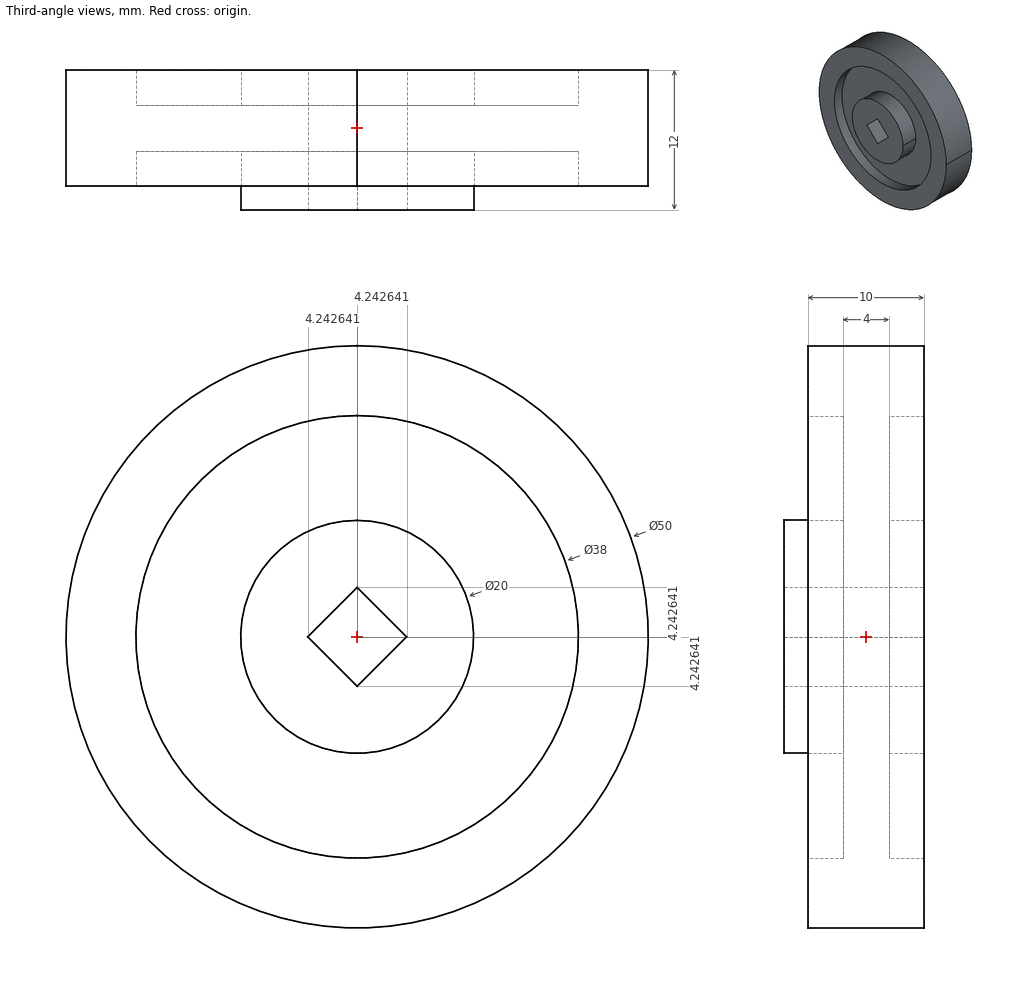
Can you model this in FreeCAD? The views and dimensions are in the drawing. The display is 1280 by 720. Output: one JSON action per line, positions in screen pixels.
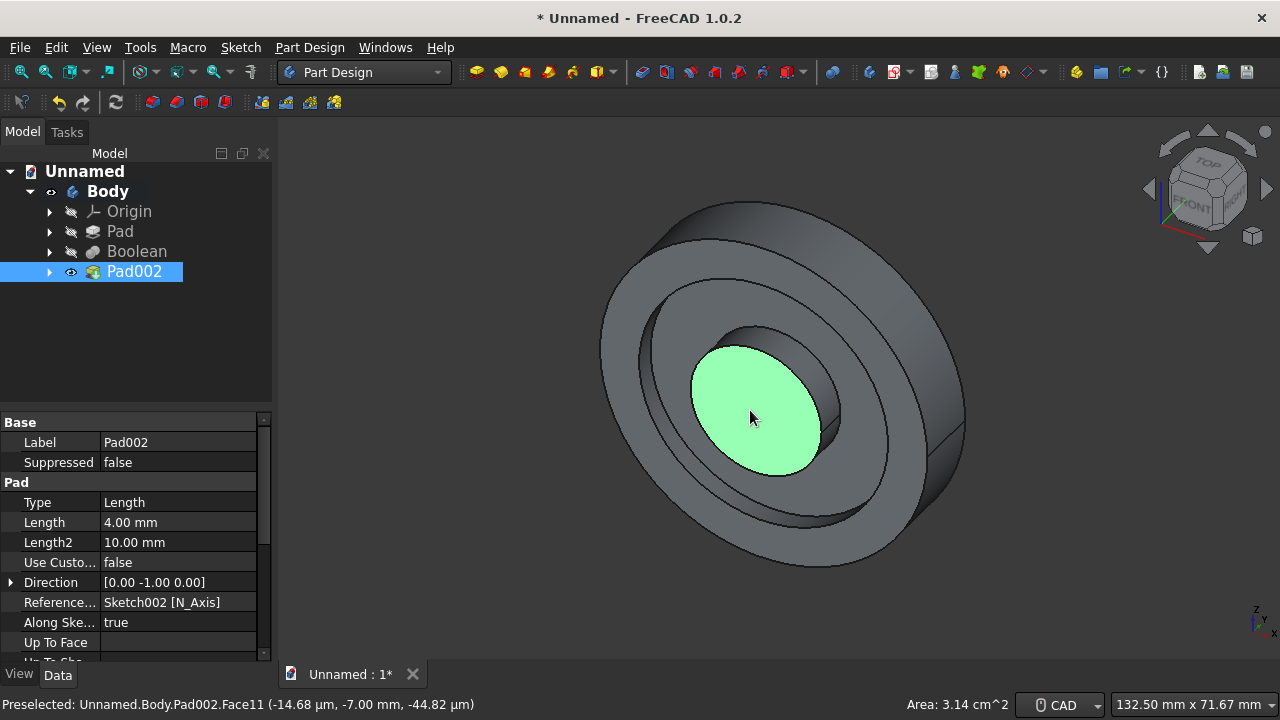
{"action": "left_click", "coordinate": [894, 72]}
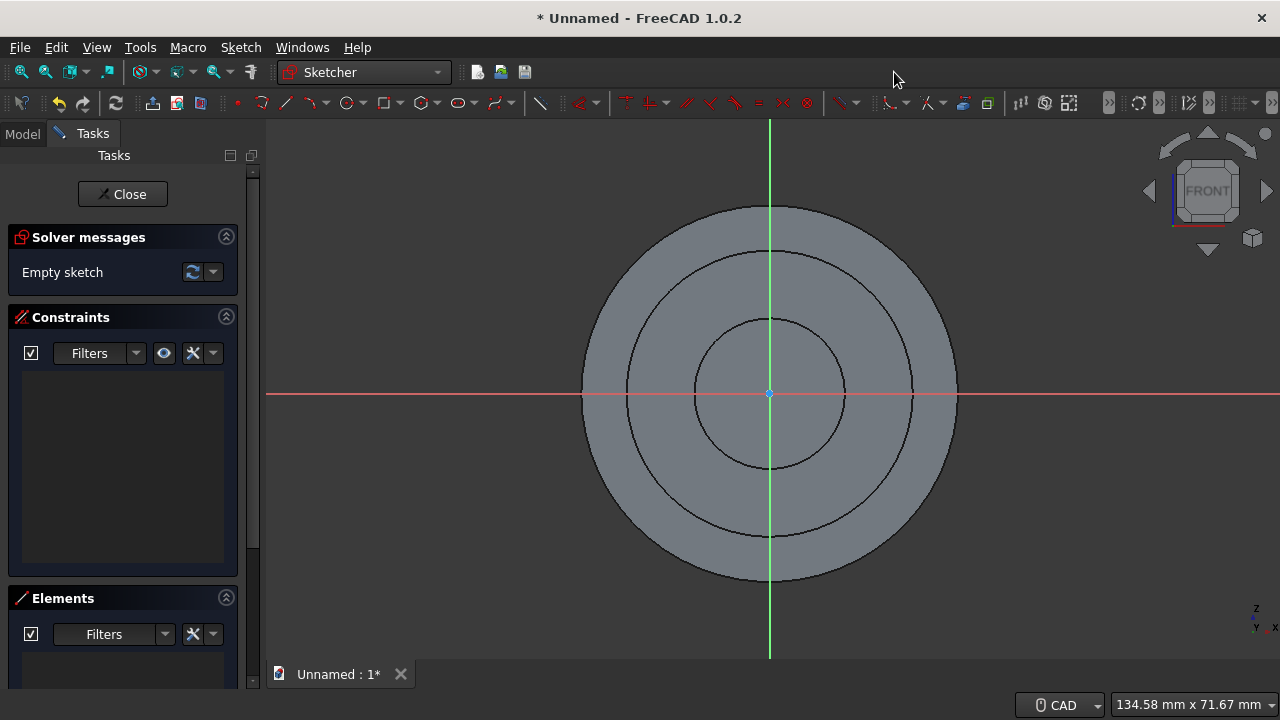
{"action": "scroll", "coordinate": [786, 395], "scroll_direction": "up", "scroll_amount": 8}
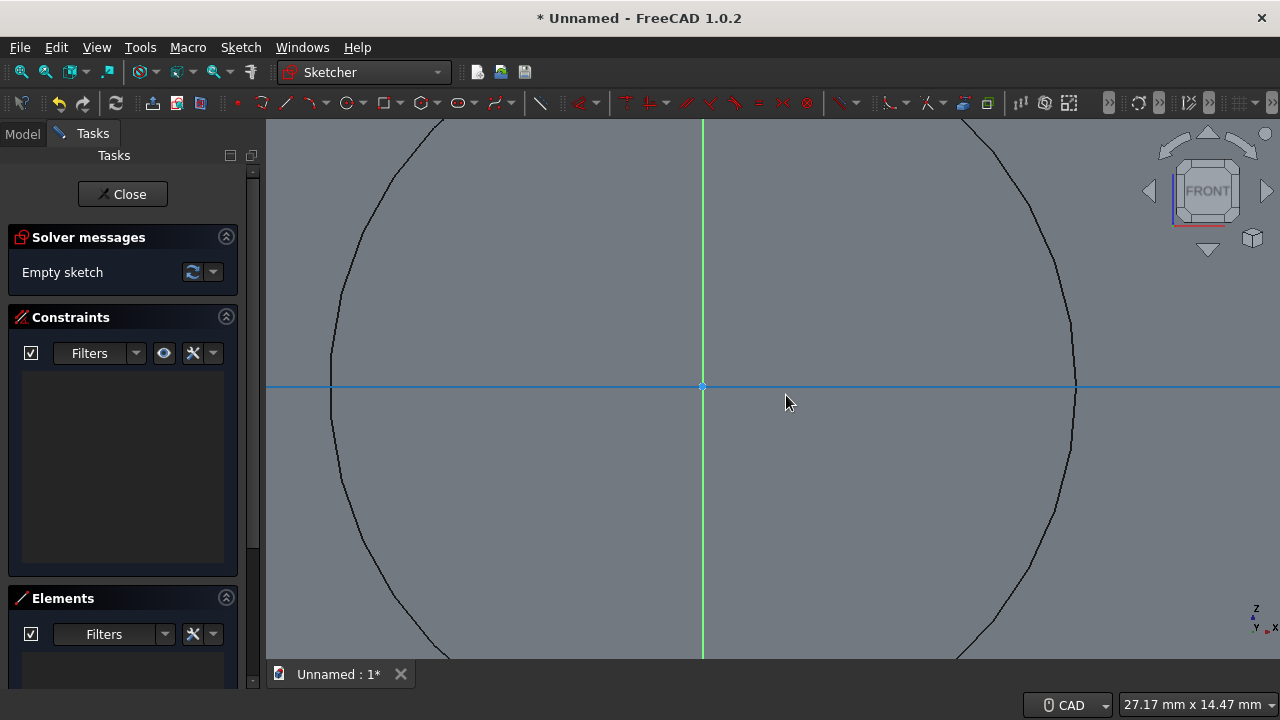
{"action": "left_click", "coordinate": [262, 104]}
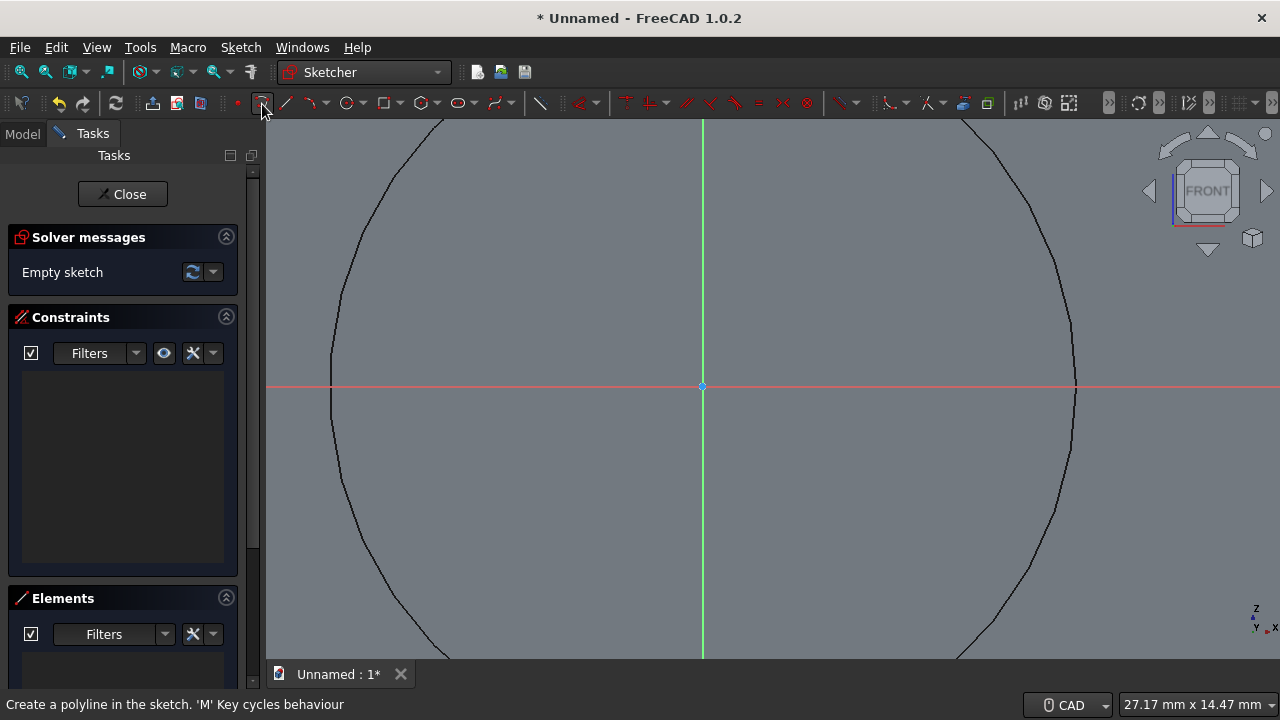
{"action": "left_click", "coordinate": [703, 228]}
{"action": "left_click", "coordinate": [545, 387]}
{"action": "left_click", "coordinate": [703, 545]}
{"action": "left_click", "coordinate": [861, 387]}
{"action": "left_click", "coordinate": [703, 229]}
{"action": "key", "text": "Escape"}
{"action": "key", "text": "Escape"}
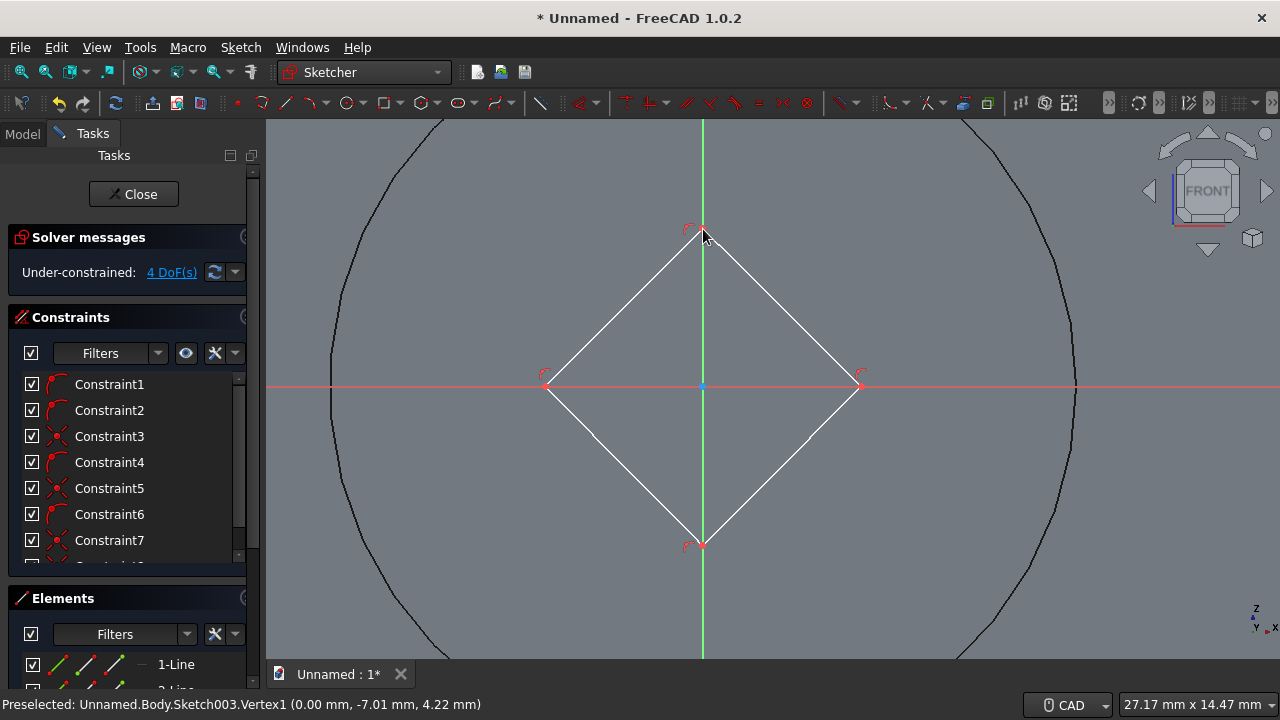
{"action": "left_click", "coordinate": [580, 104]}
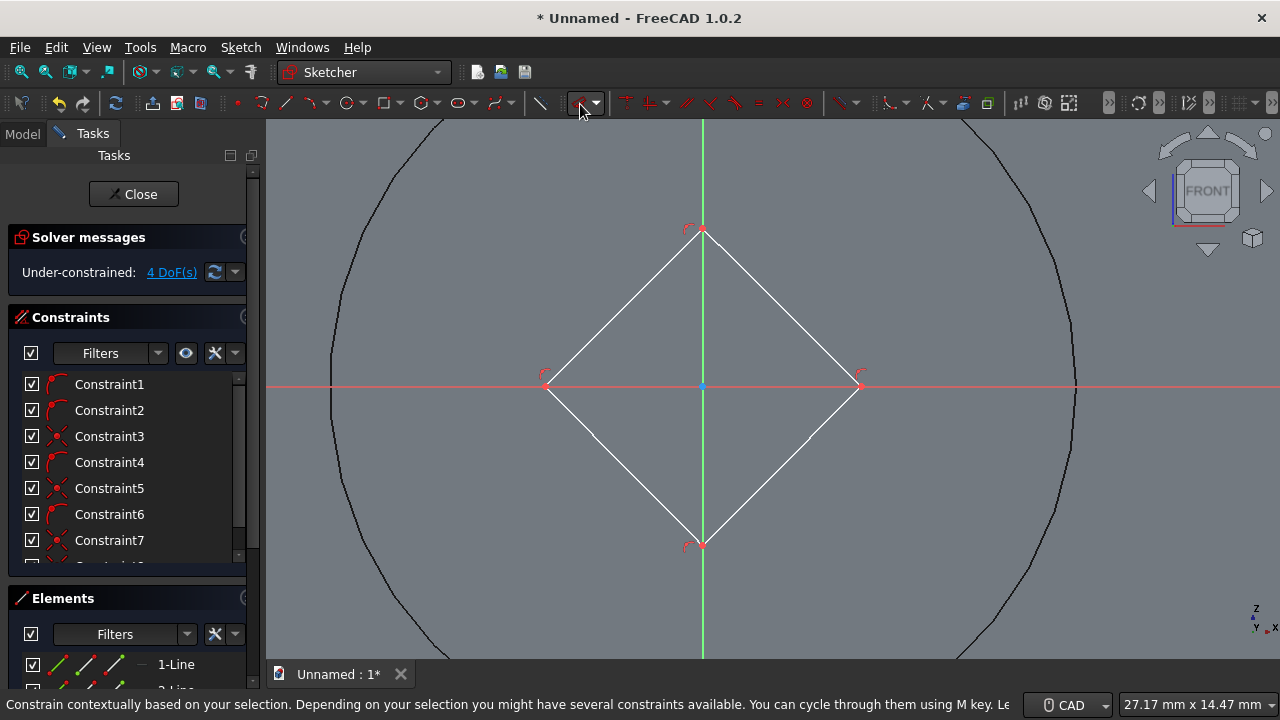
{"action": "left_click", "coordinate": [703, 229]}
{"action": "left_click", "coordinate": [737, 308]}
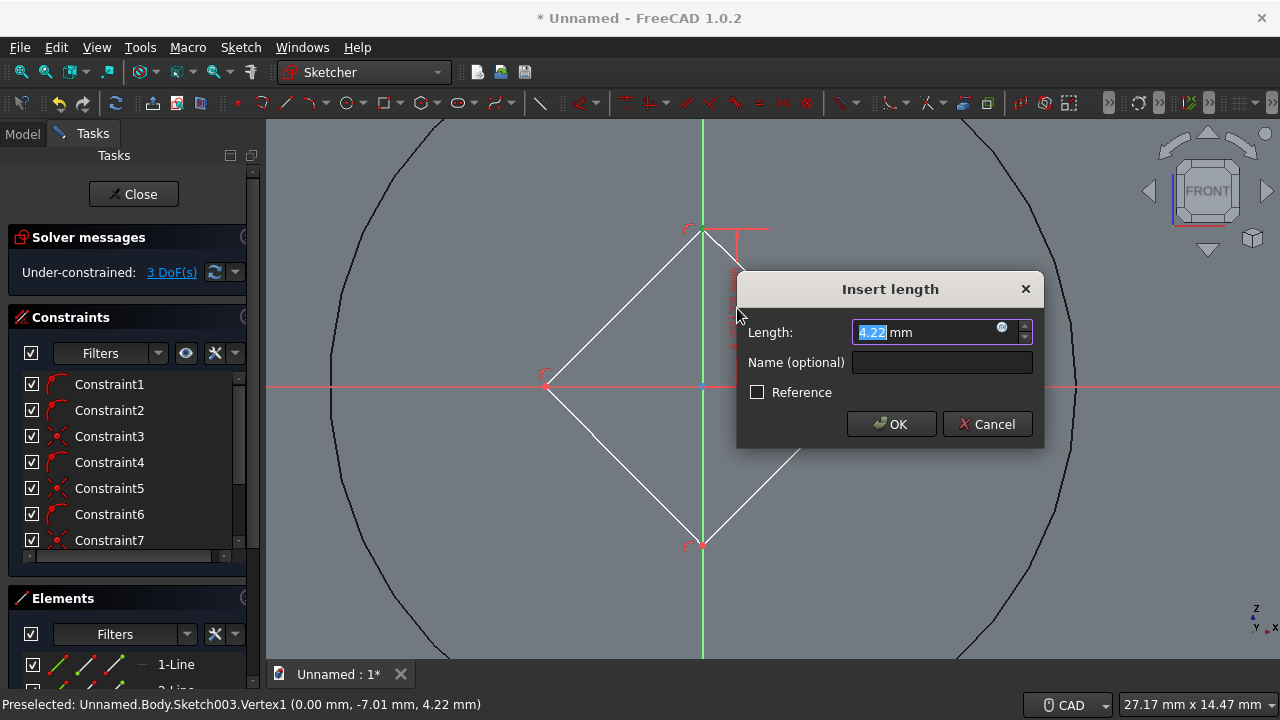
{"action": "type", "text": "4.242641"}
{"action": "key", "text": "Return"}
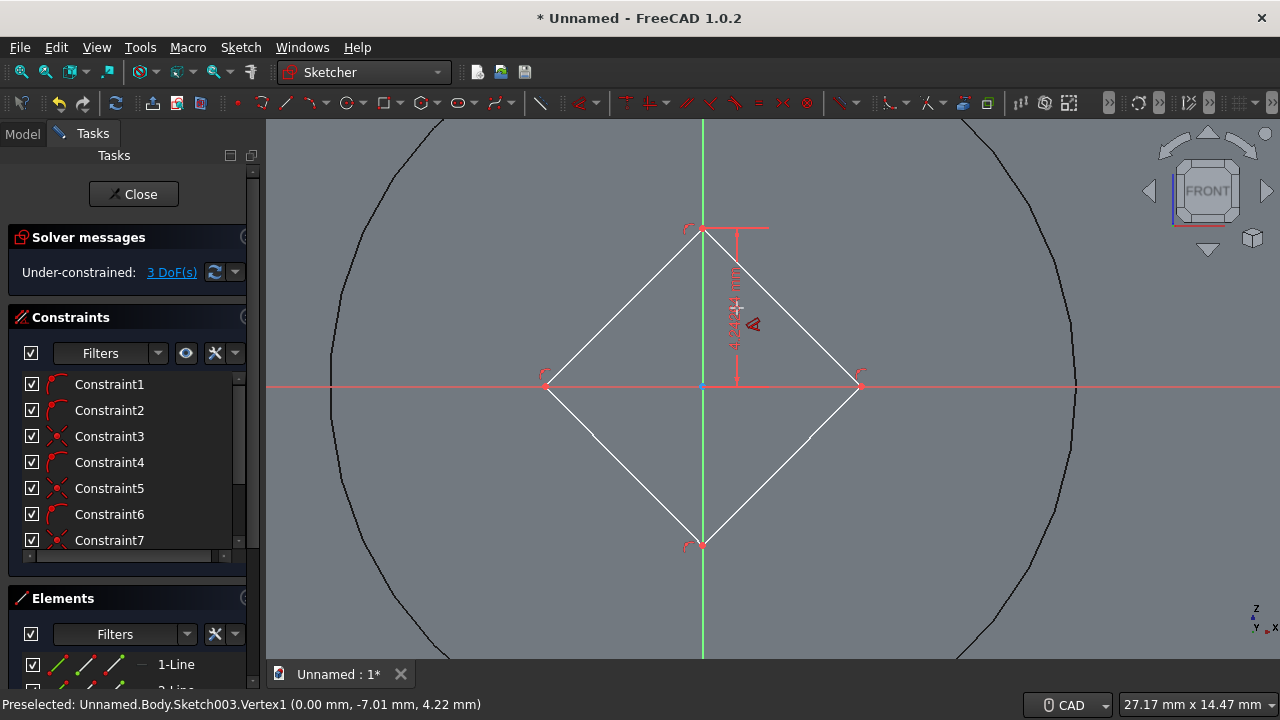
{"action": "left_click", "coordinate": [545, 387]}
{"action": "left_click", "coordinate": [624, 421]}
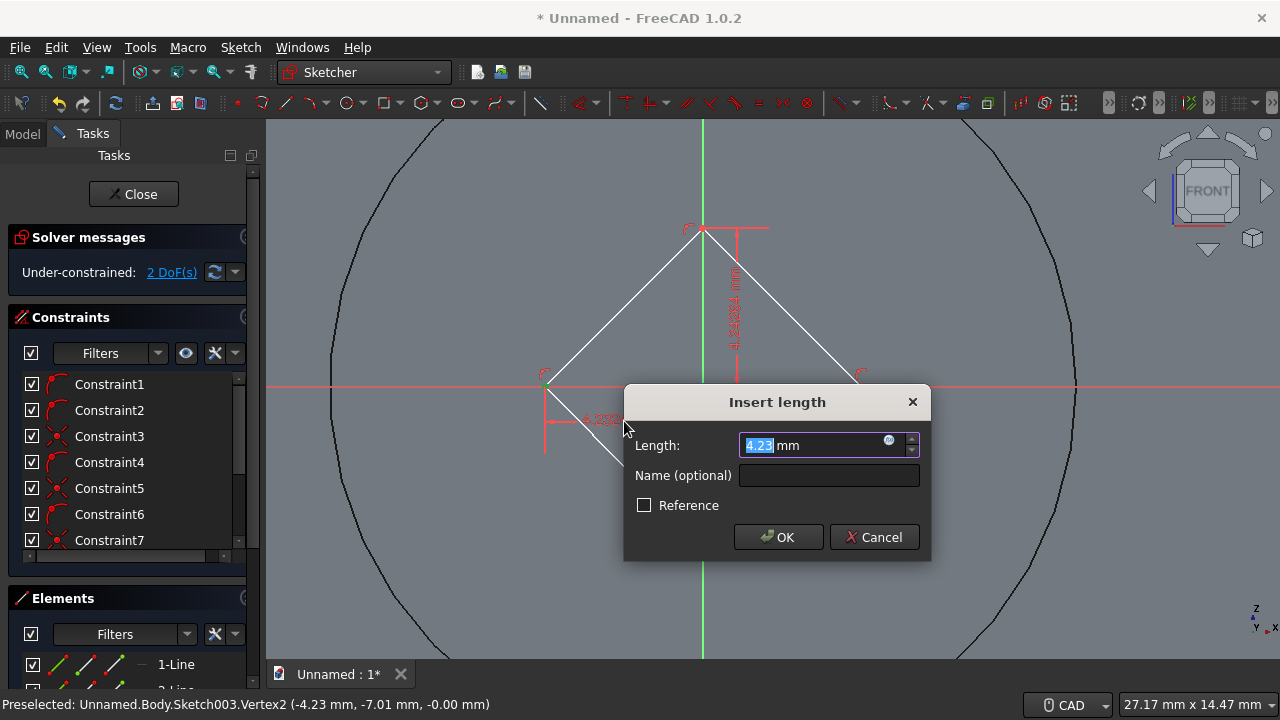
{"action": "type", "text": "4.242641"}
{"action": "key", "text": "Return"}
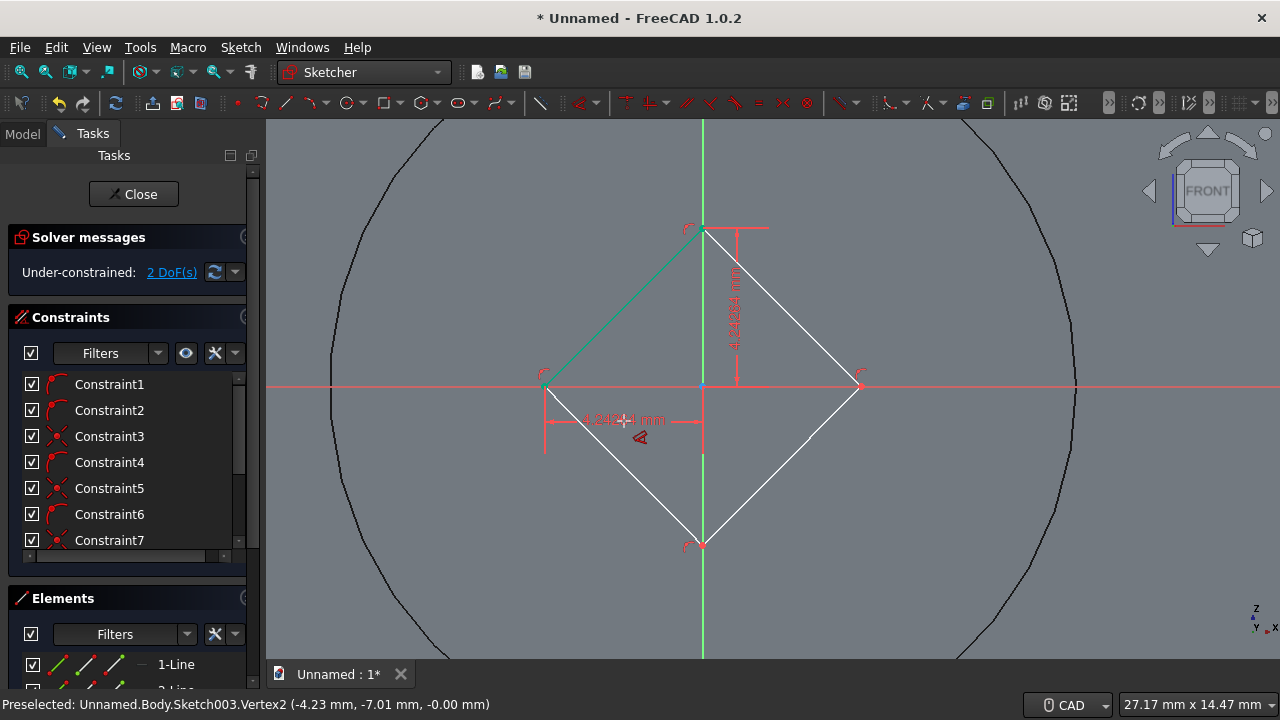
{"action": "left_click", "coordinate": [703, 546]}
{"action": "left_click", "coordinate": [737, 466]}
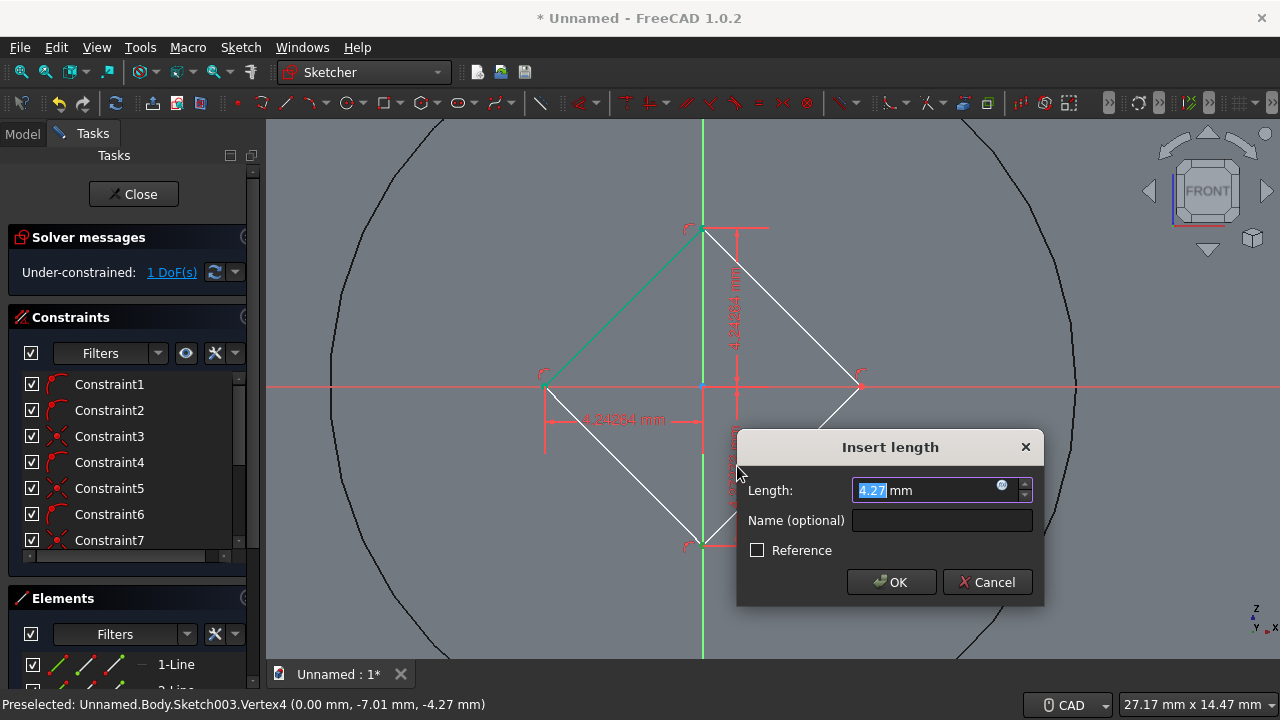
{"action": "type", "text": "4.242641"}
{"action": "key", "text": "Return"}